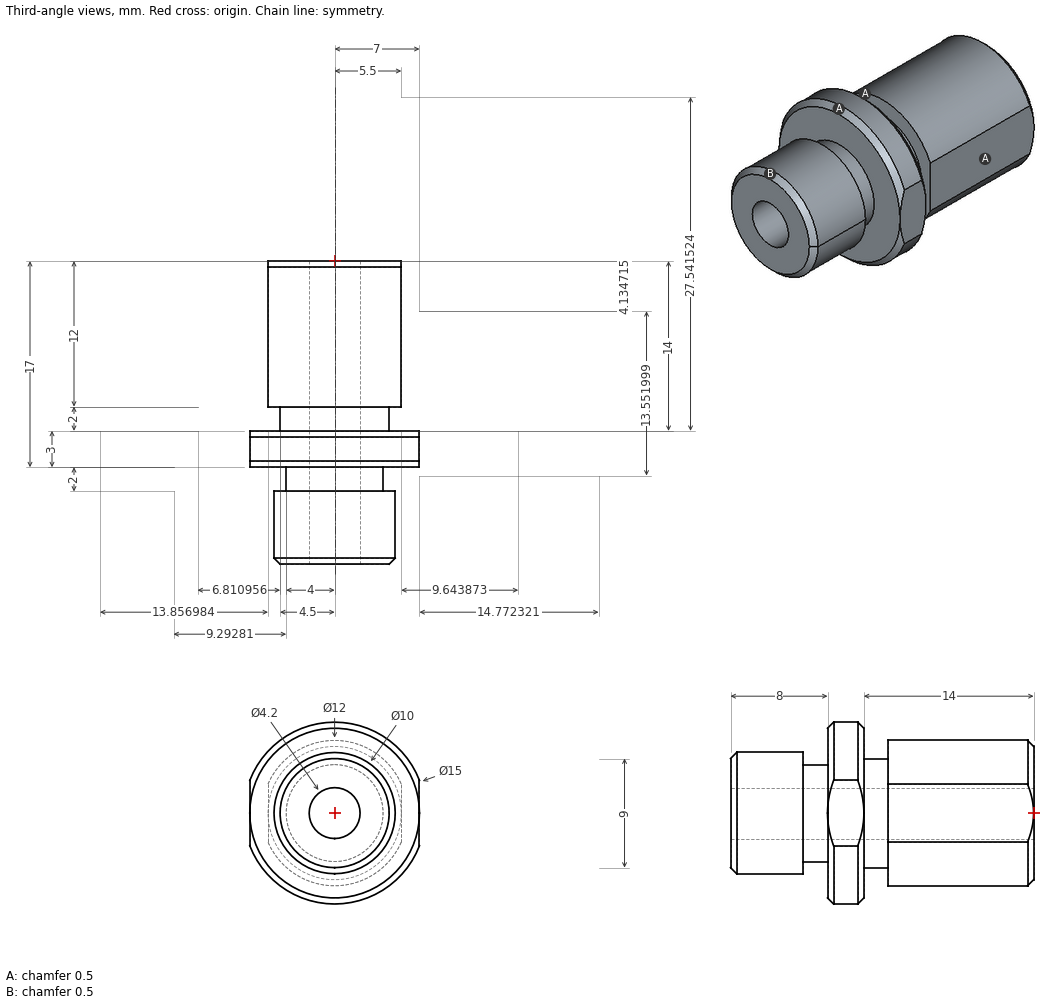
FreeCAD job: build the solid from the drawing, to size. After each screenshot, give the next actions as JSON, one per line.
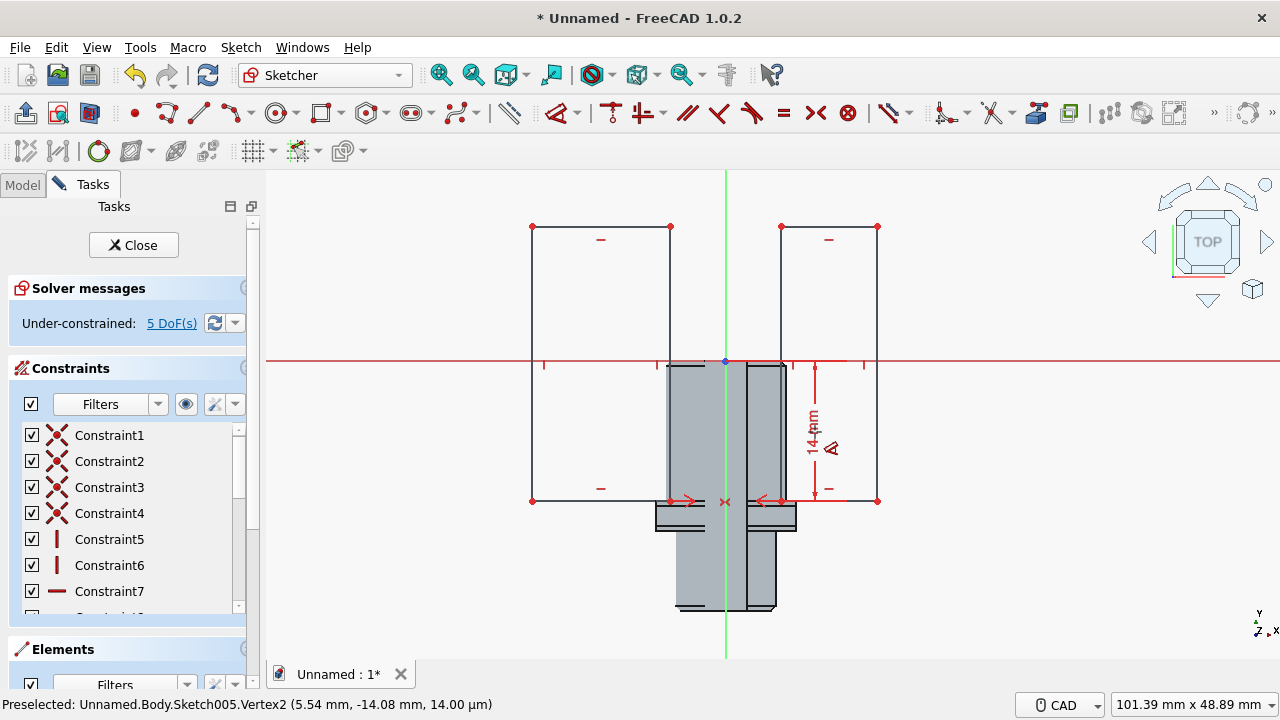
{"action": "left_click", "coordinate": [781, 227]}
{"action": "left_click", "coordinate": [753, 395]}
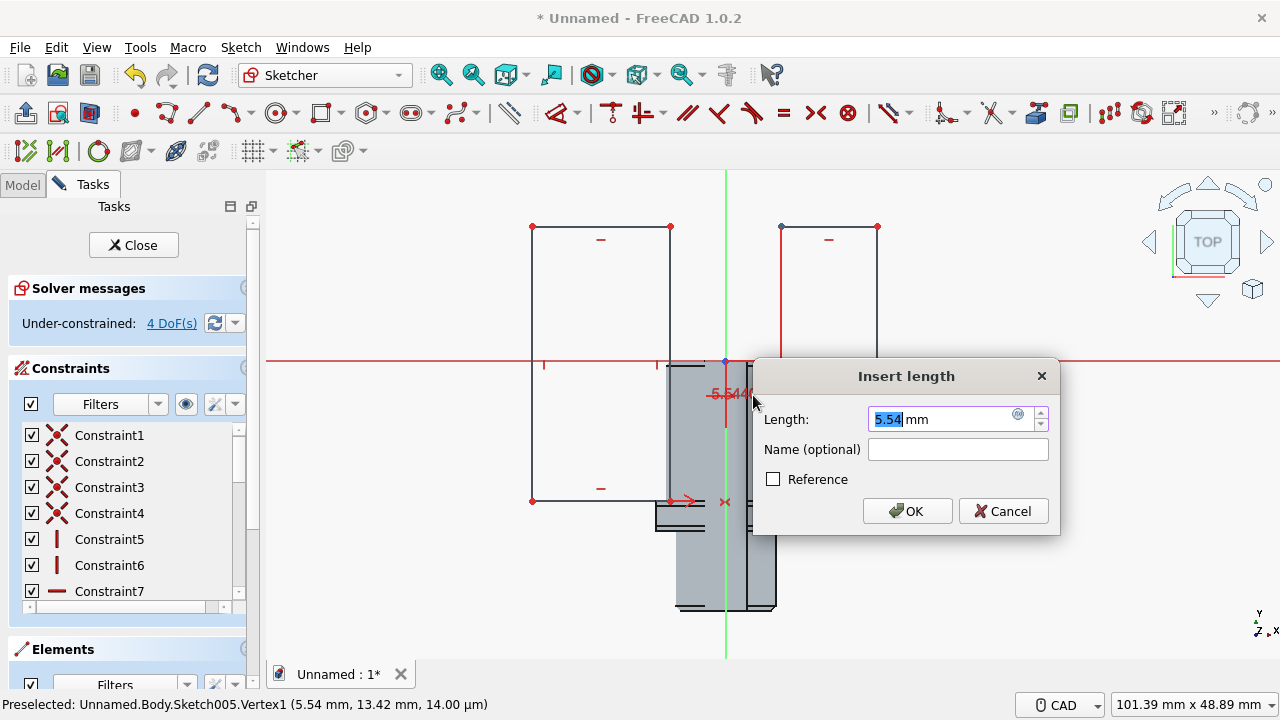
{"action": "type", "text": "5.5"}
{"action": "key", "text": "Return"}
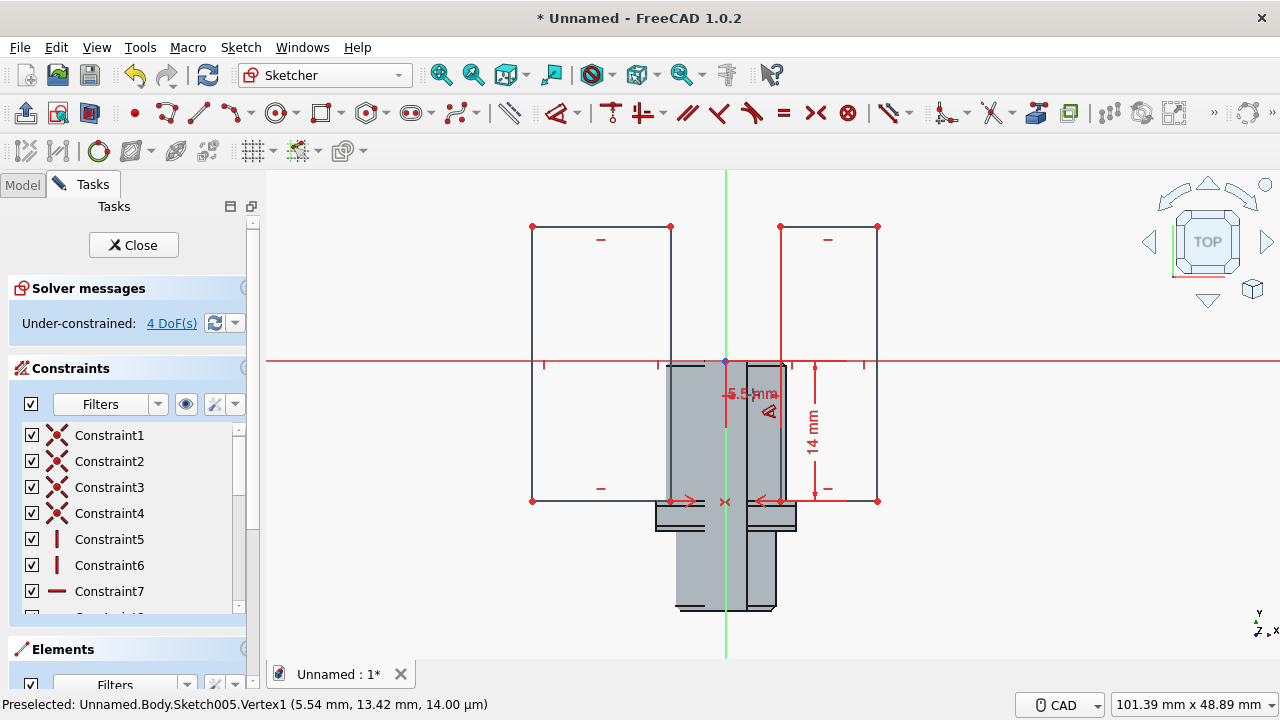
{"action": "left_click", "coordinate": [809, 501]}
{"action": "left_click", "coordinate": [829, 535]}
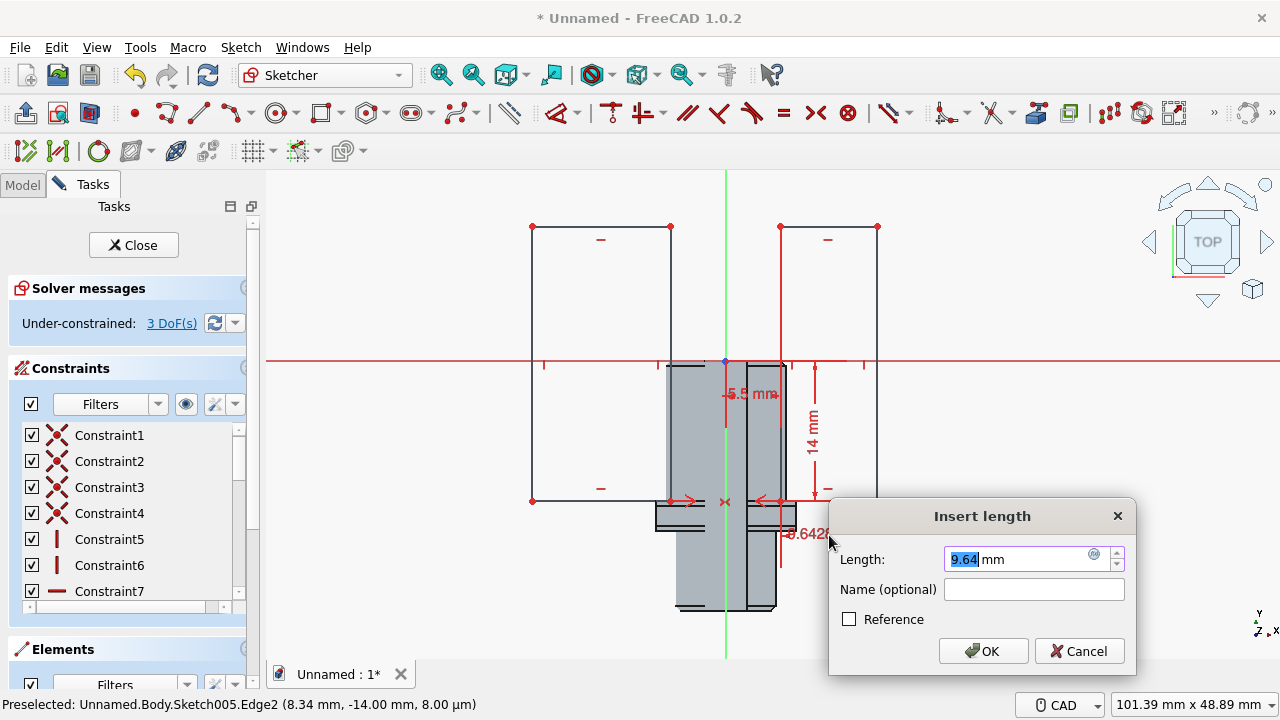
{"action": "type", "text": "9.643873"}
{"action": "key", "text": "Return"}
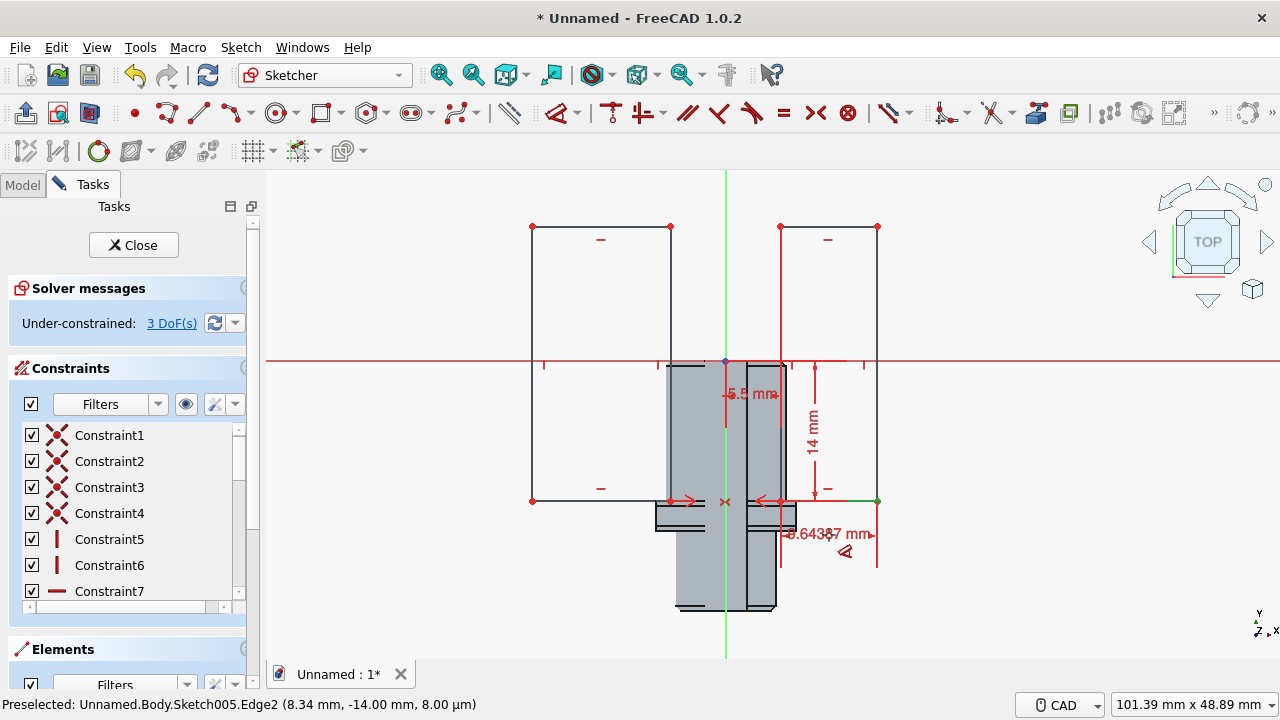
{"action": "left_click", "coordinate": [781, 309]}
{"action": "left_click", "coordinate": [815, 301]}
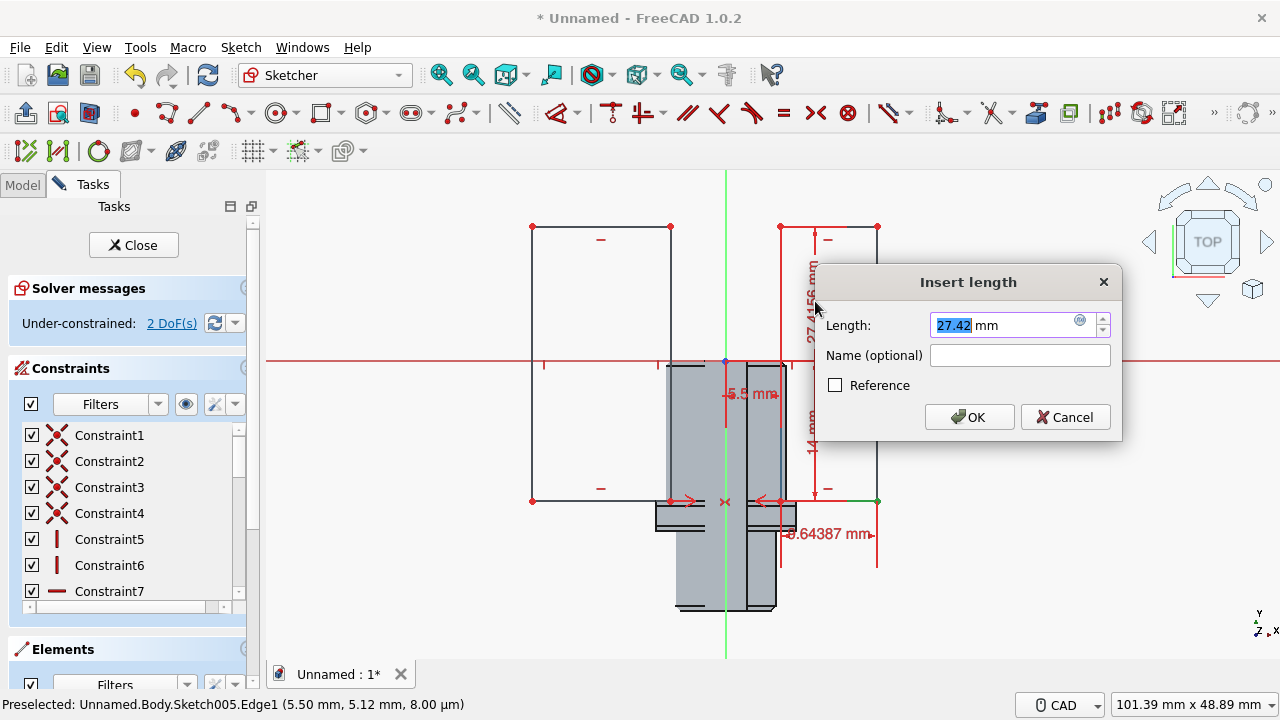
{"action": "type", "text": "27.541524"}
{"action": "key", "text": "Return"}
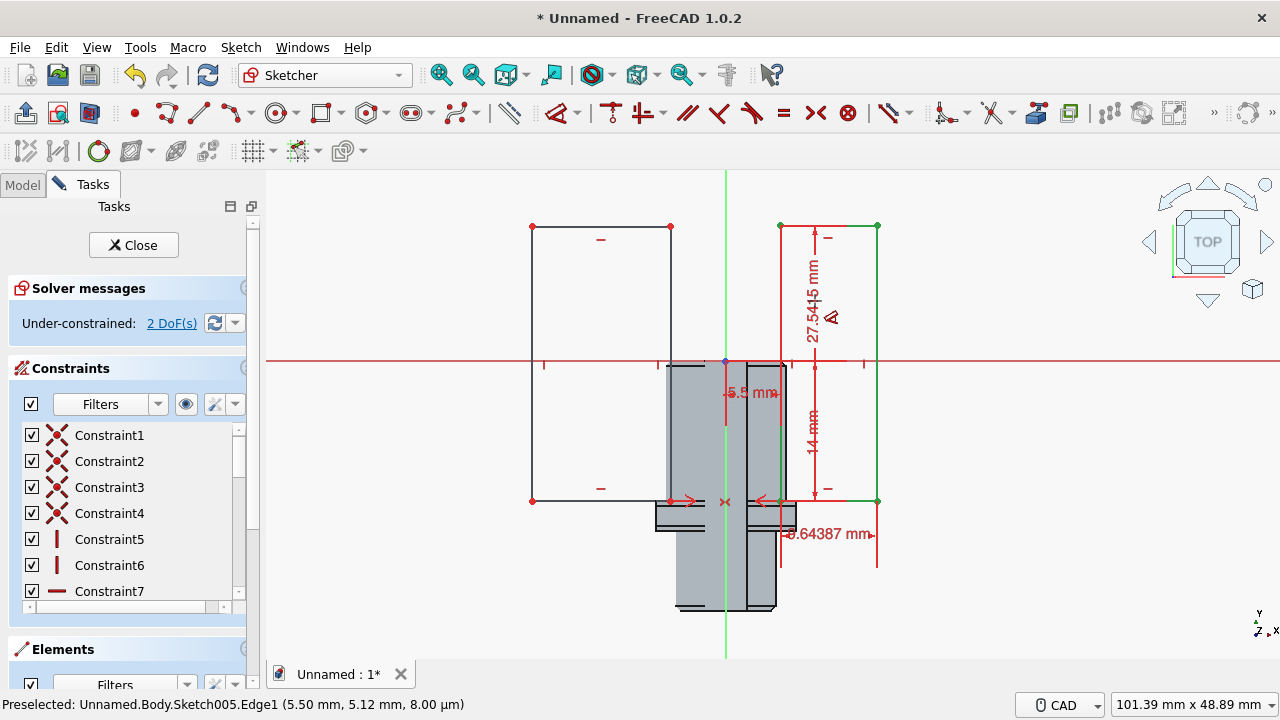
{"action": "left_click", "coordinate": [532, 309]}
{"action": "left_click", "coordinate": [498, 301]}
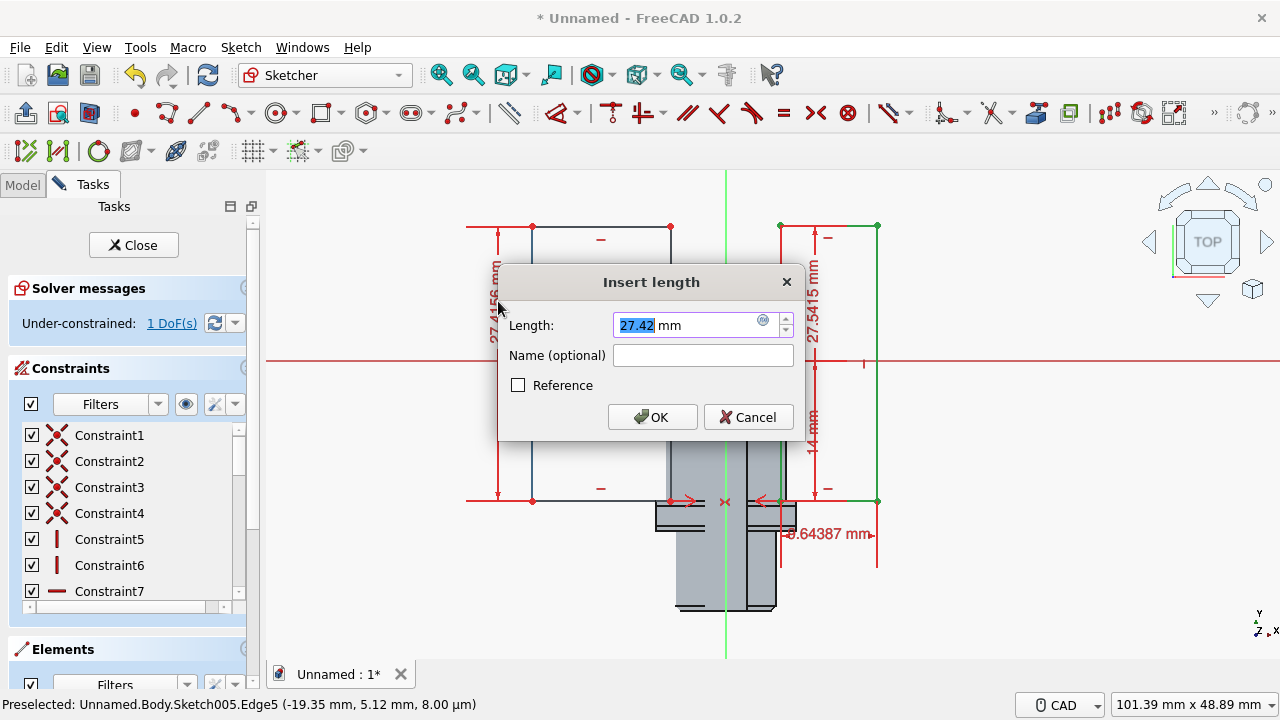
{"action": "type", "text": "27.541524"}
{"action": "key", "text": "Return"}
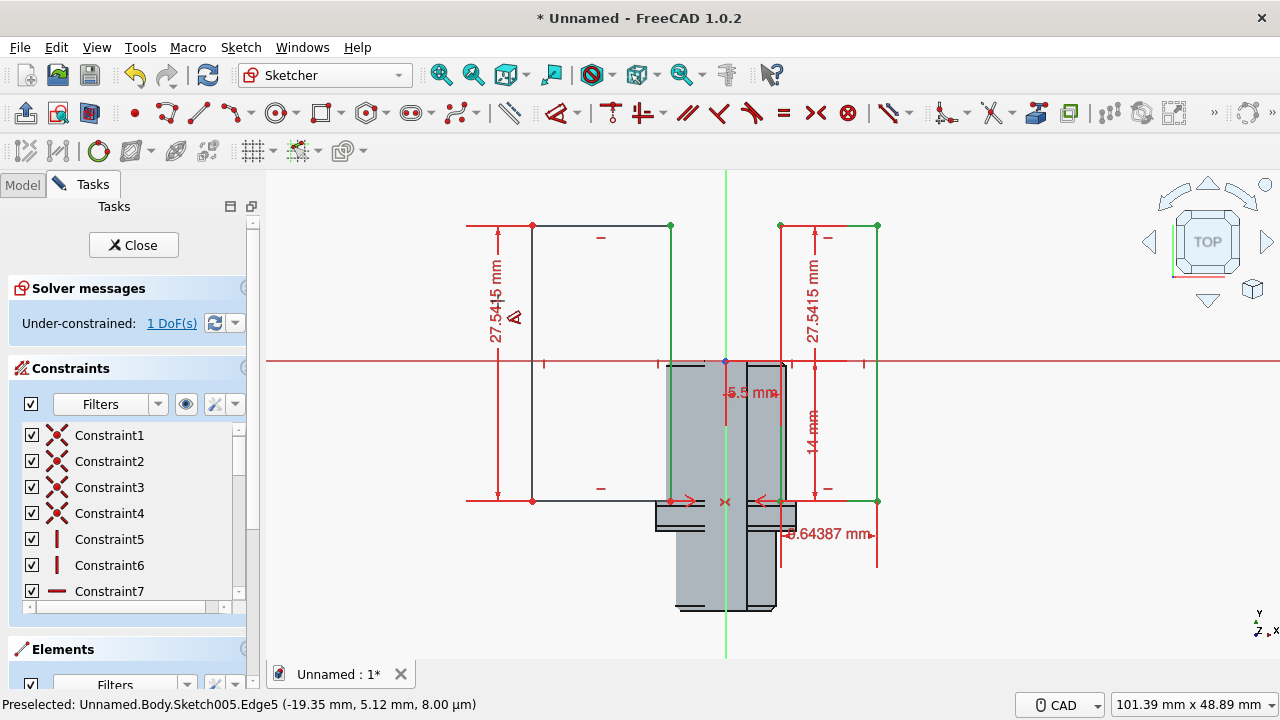
{"action": "left_click", "coordinate": [574, 501]}
{"action": "left_click", "coordinate": [601, 535]}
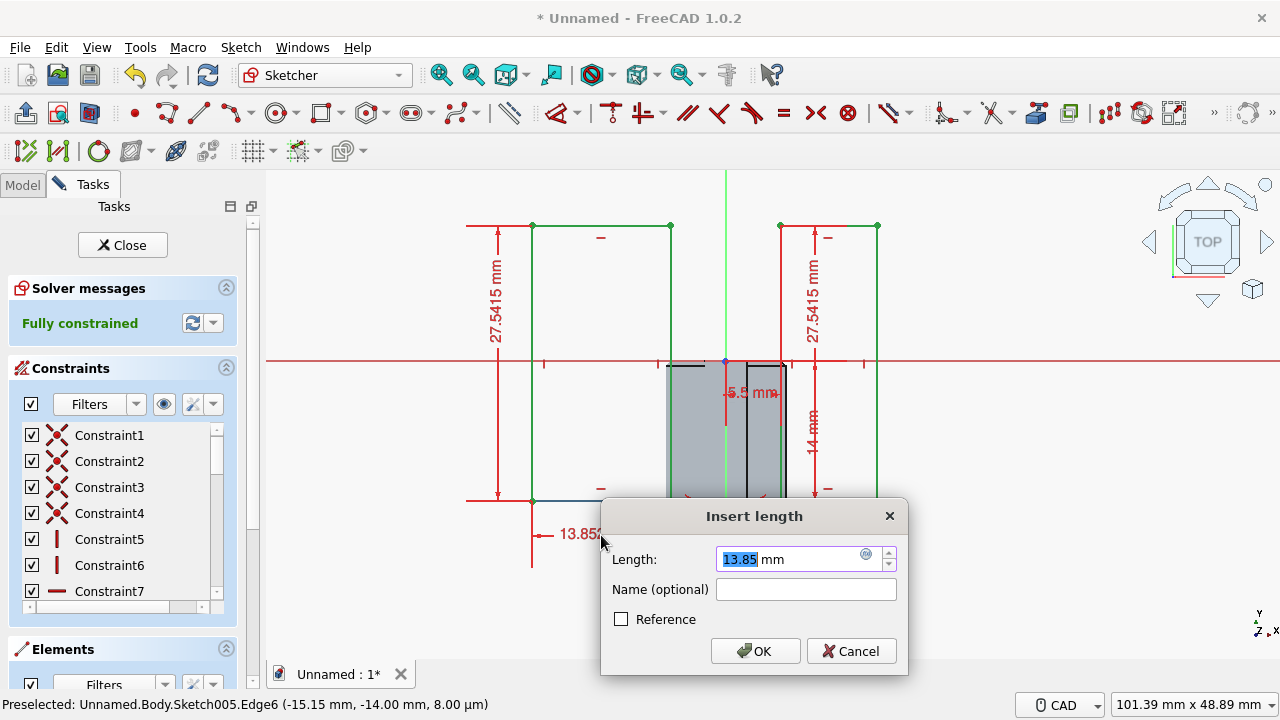
{"action": "type", "text": "13.856984"}
{"action": "key", "text": "Return"}
{"action": "key", "text": "Escape"}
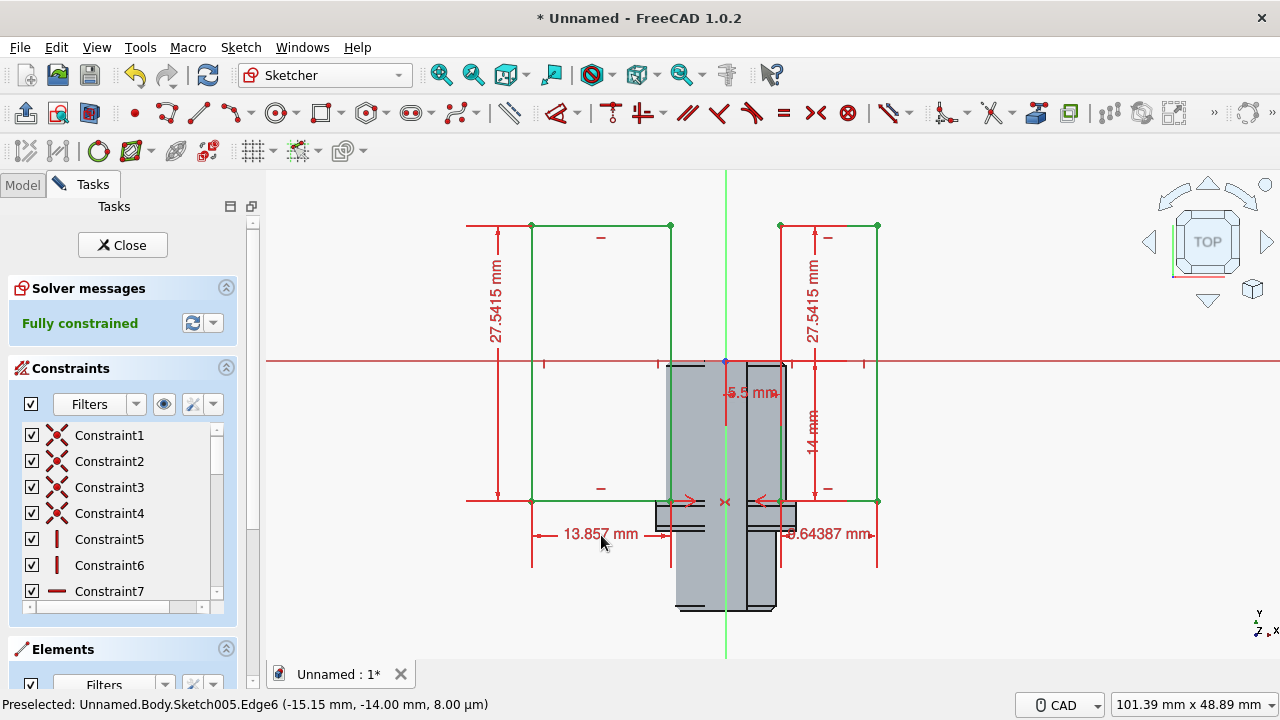
{"action": "left_click", "coordinate": [123, 245]}